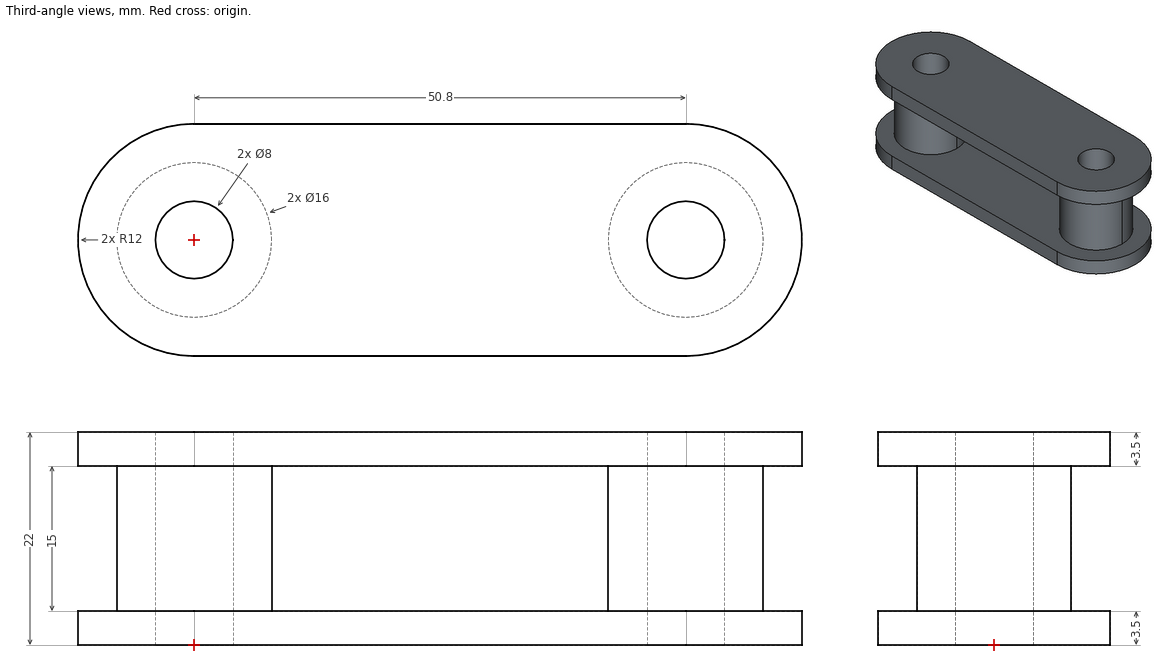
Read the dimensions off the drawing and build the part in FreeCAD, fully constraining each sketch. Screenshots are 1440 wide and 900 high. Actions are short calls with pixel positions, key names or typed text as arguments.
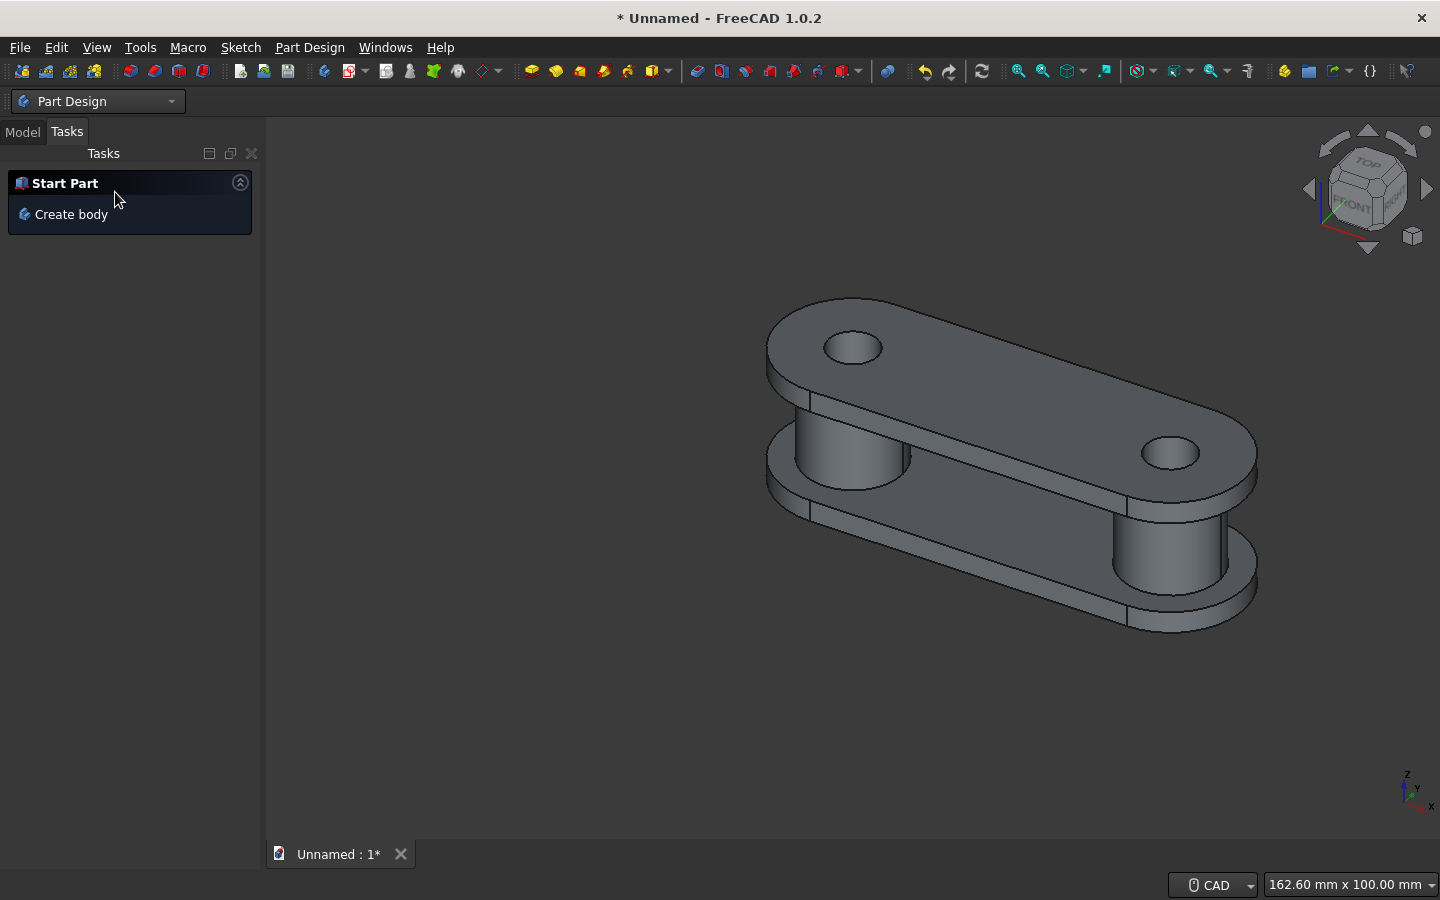
key(0)